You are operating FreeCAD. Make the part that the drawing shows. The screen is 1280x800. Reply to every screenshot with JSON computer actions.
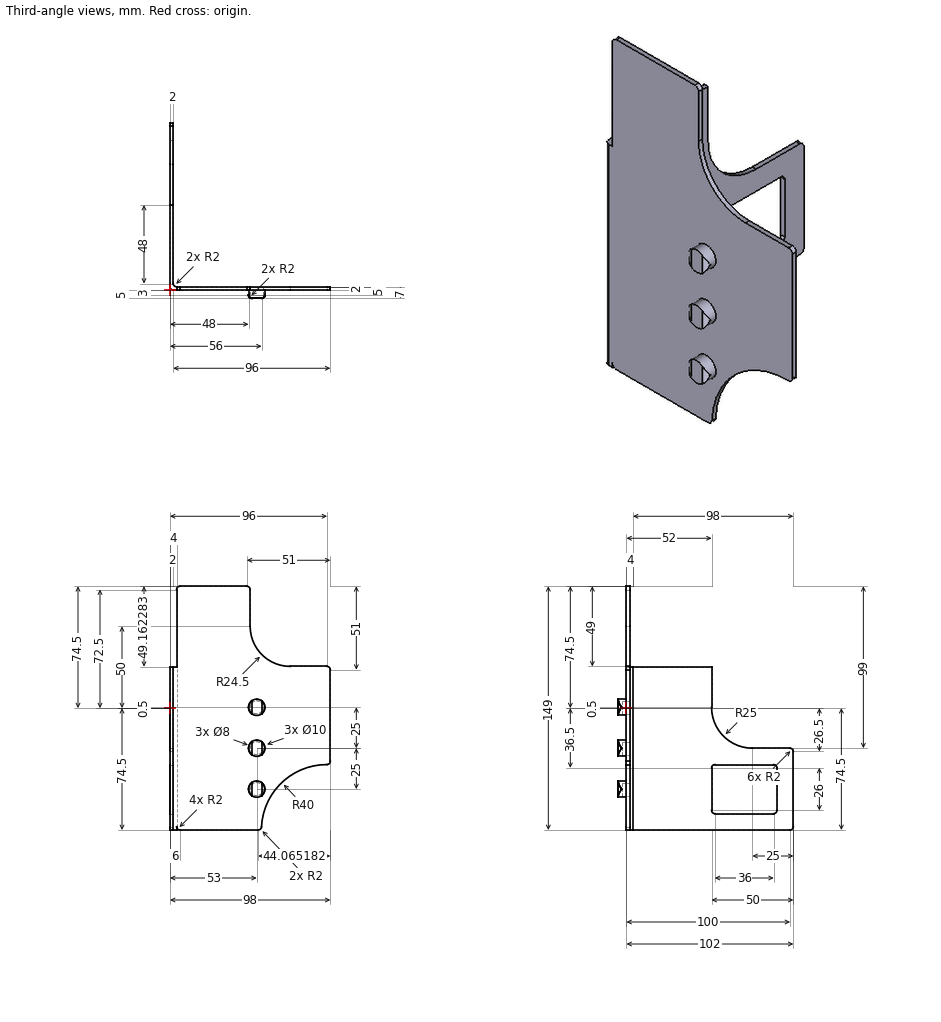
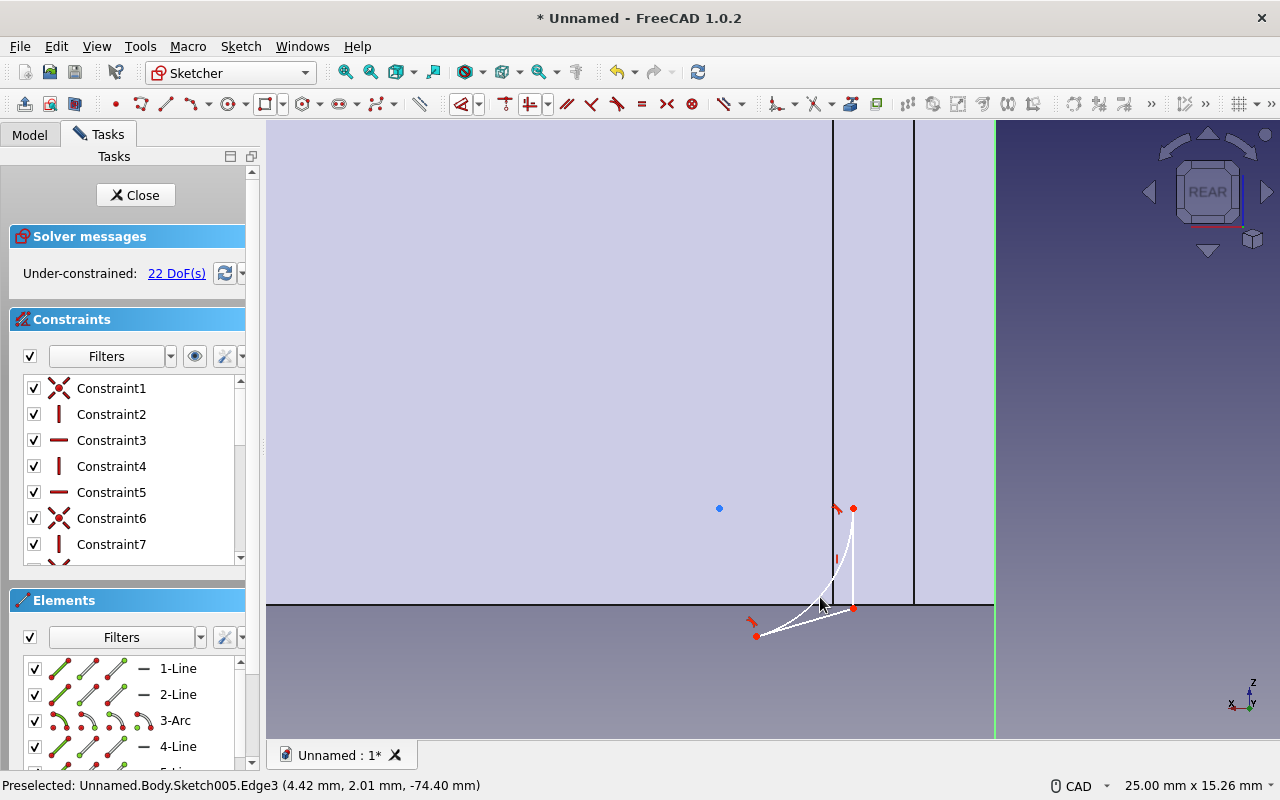
{"action": "scroll", "coordinate": [814, 614], "scroll_direction": "down", "scroll_amount": 14}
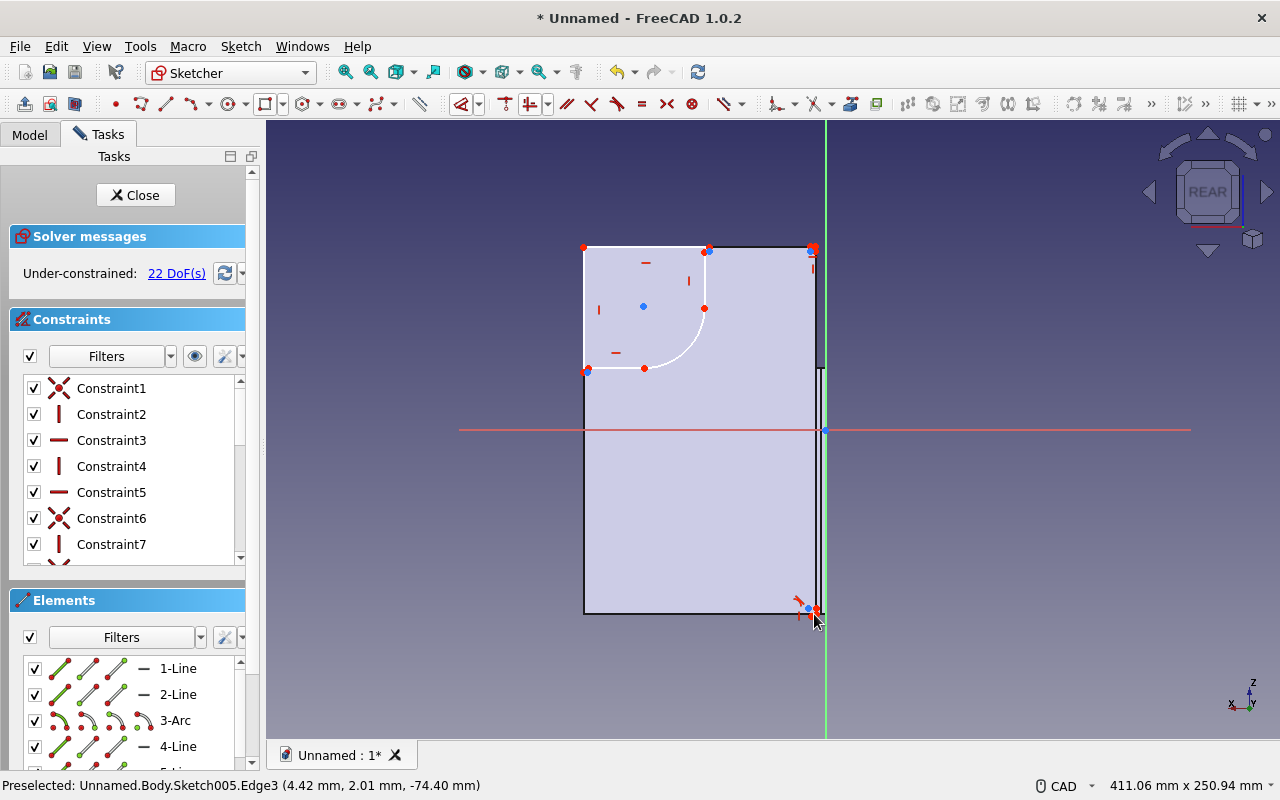
{"action": "left_click", "coordinate": [605, 368]}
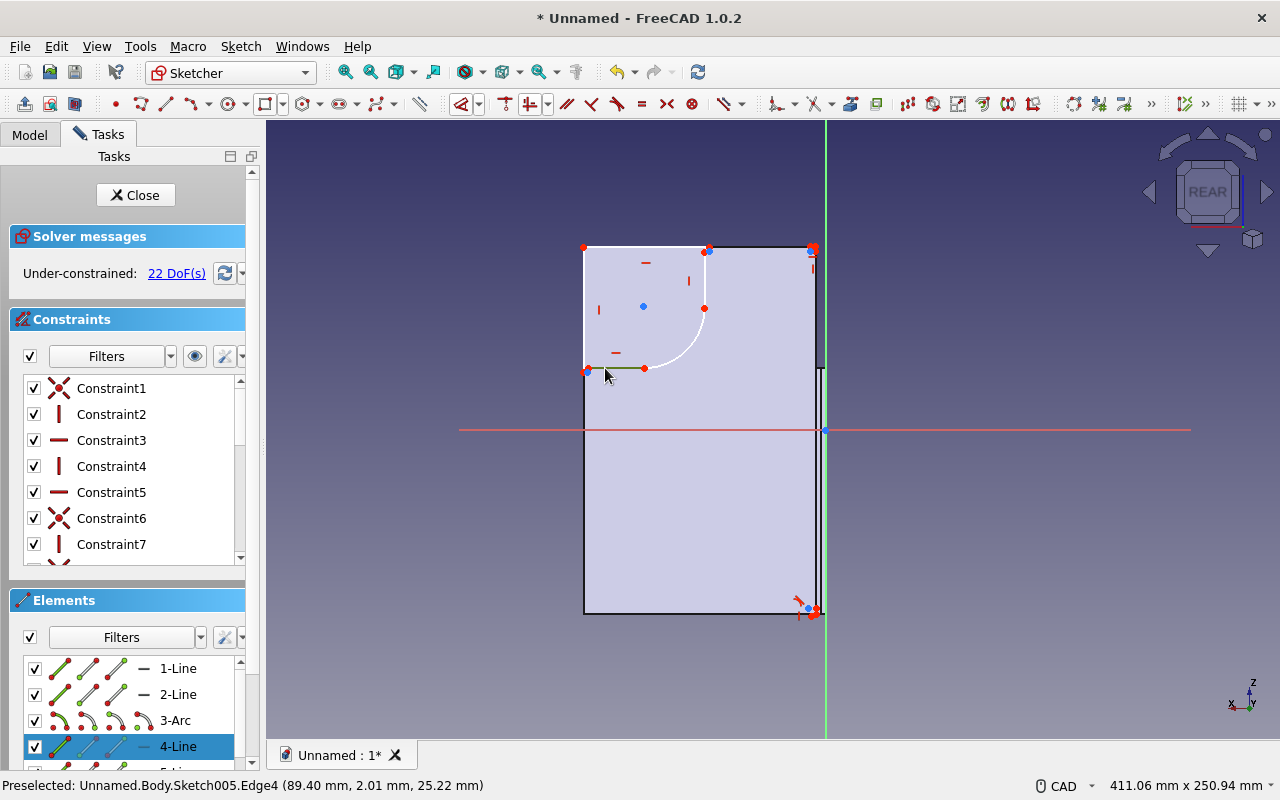
{"action": "left_click", "coordinate": [672, 361]}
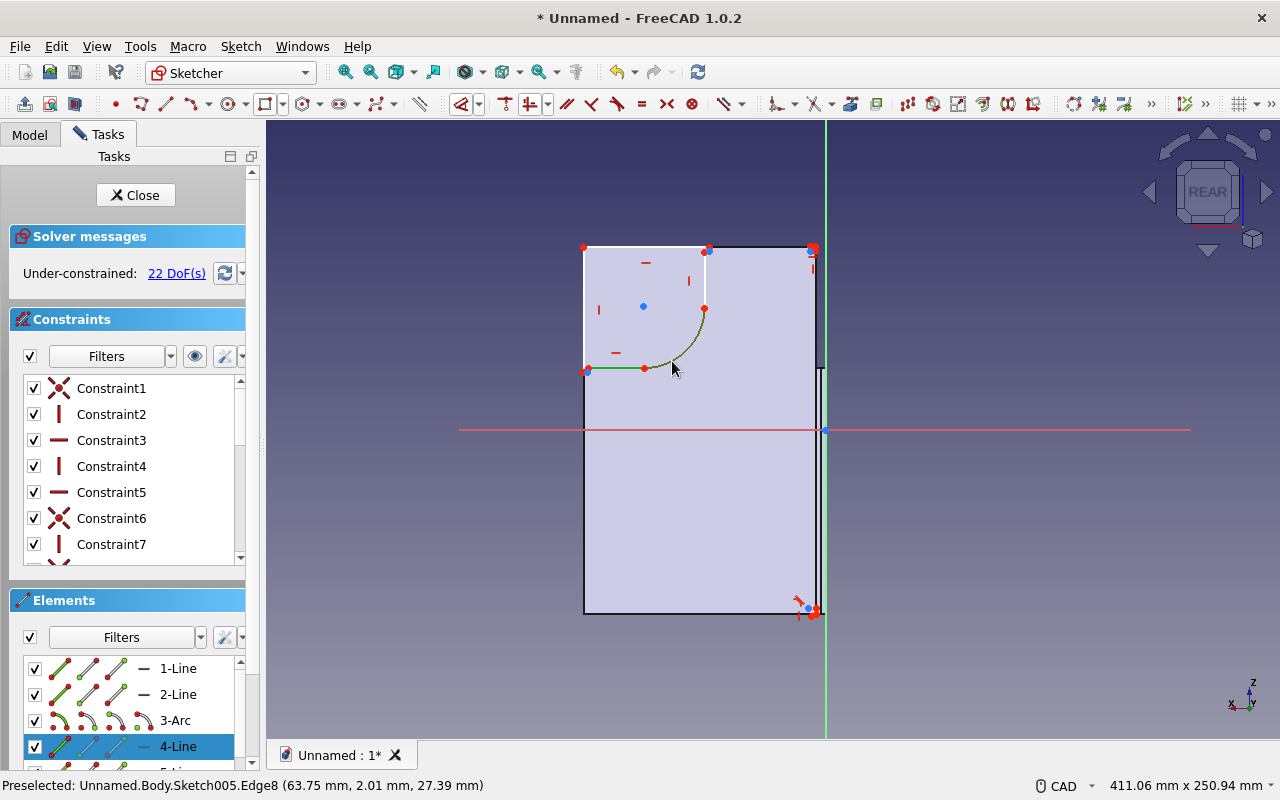
{"action": "key", "text": "t"}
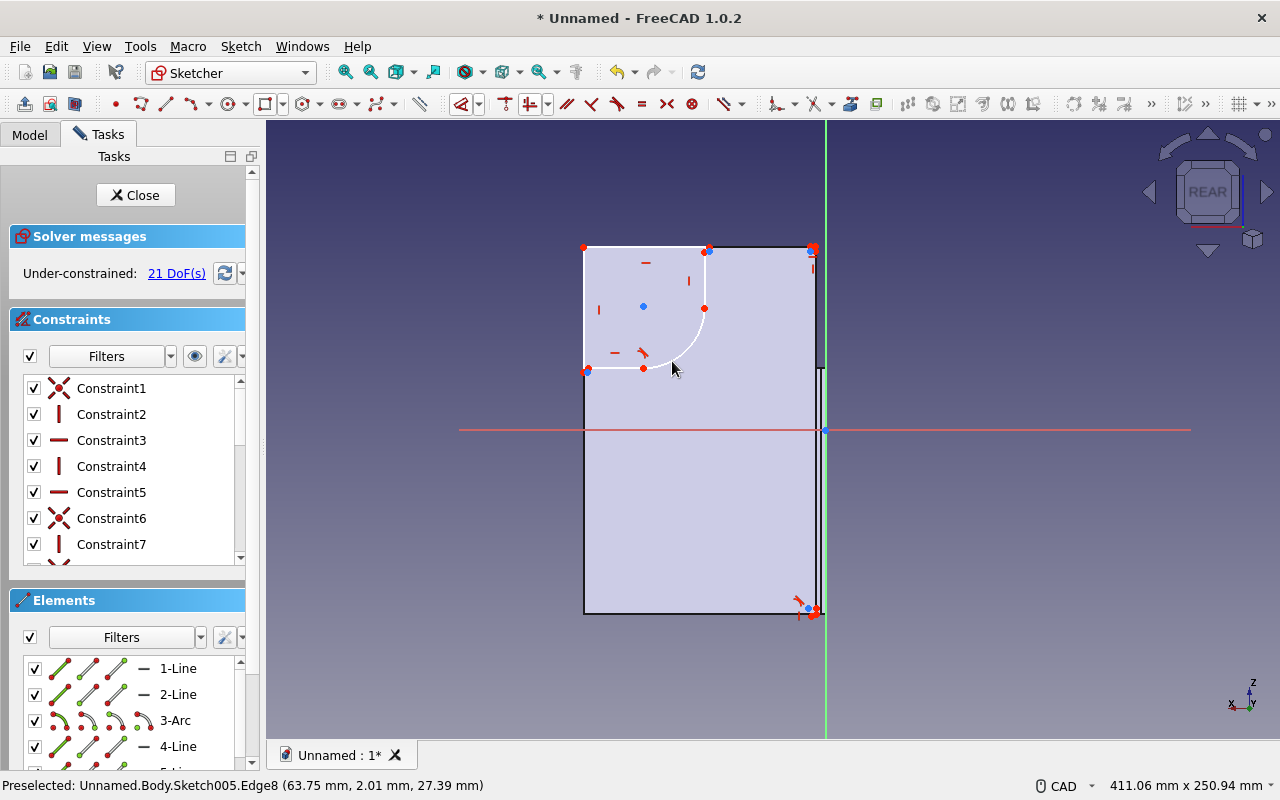
{"action": "left_click", "coordinate": [605, 368]}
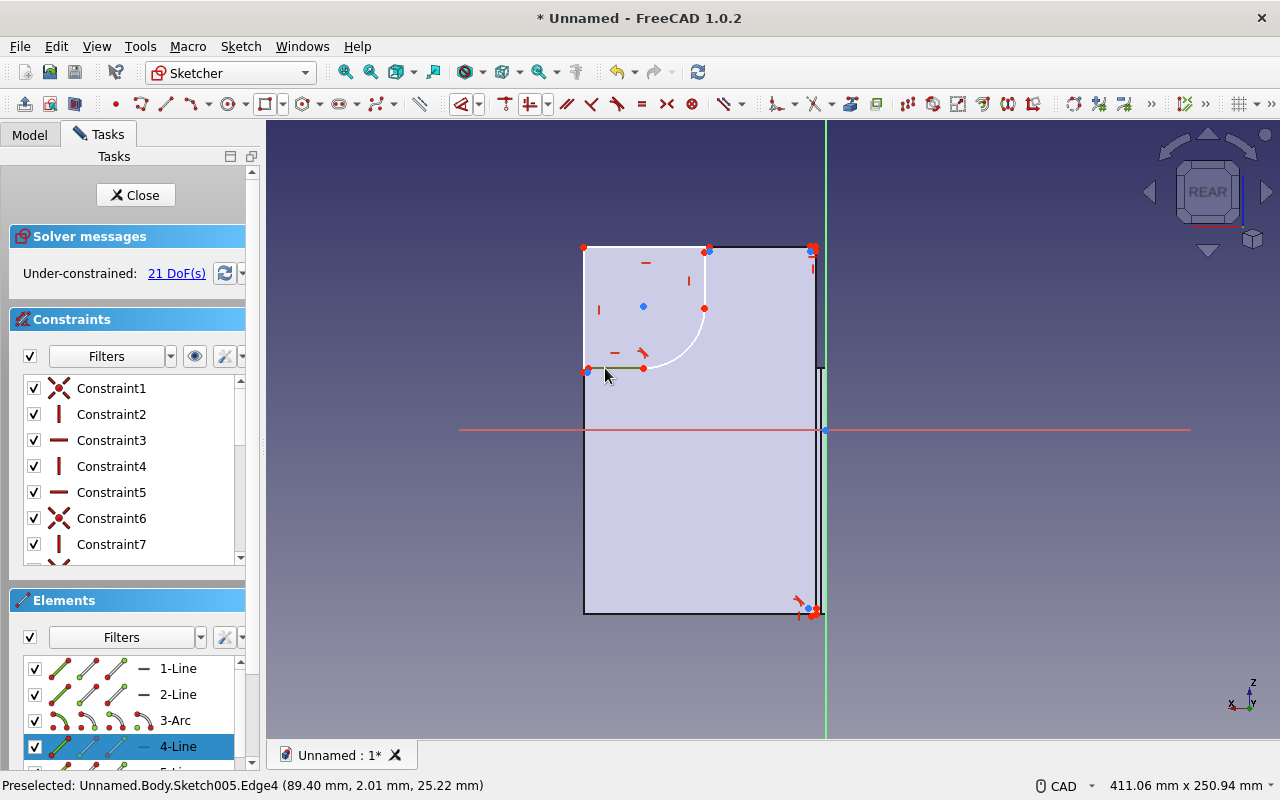
{"action": "scroll", "coordinate": [586, 368], "scroll_direction": "up", "scroll_amount": 9}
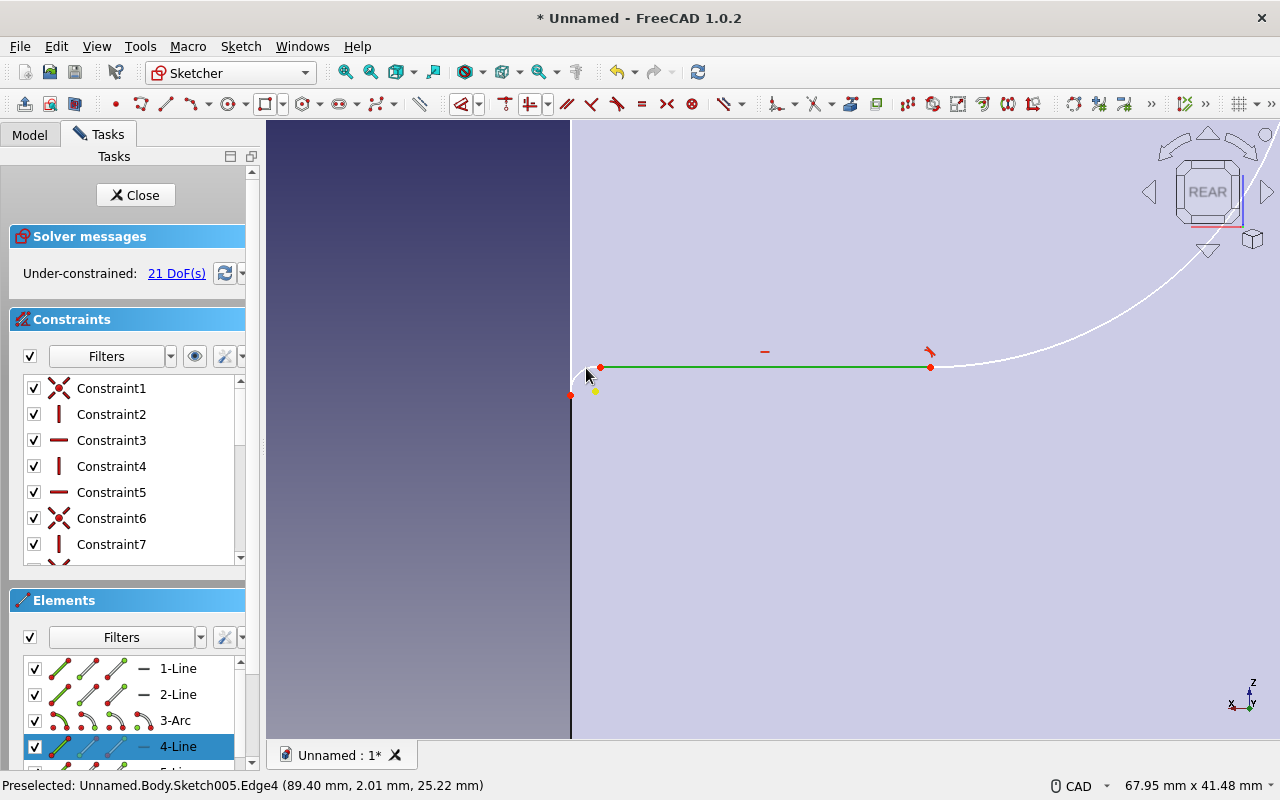
{"action": "left_click", "coordinate": [586, 369]}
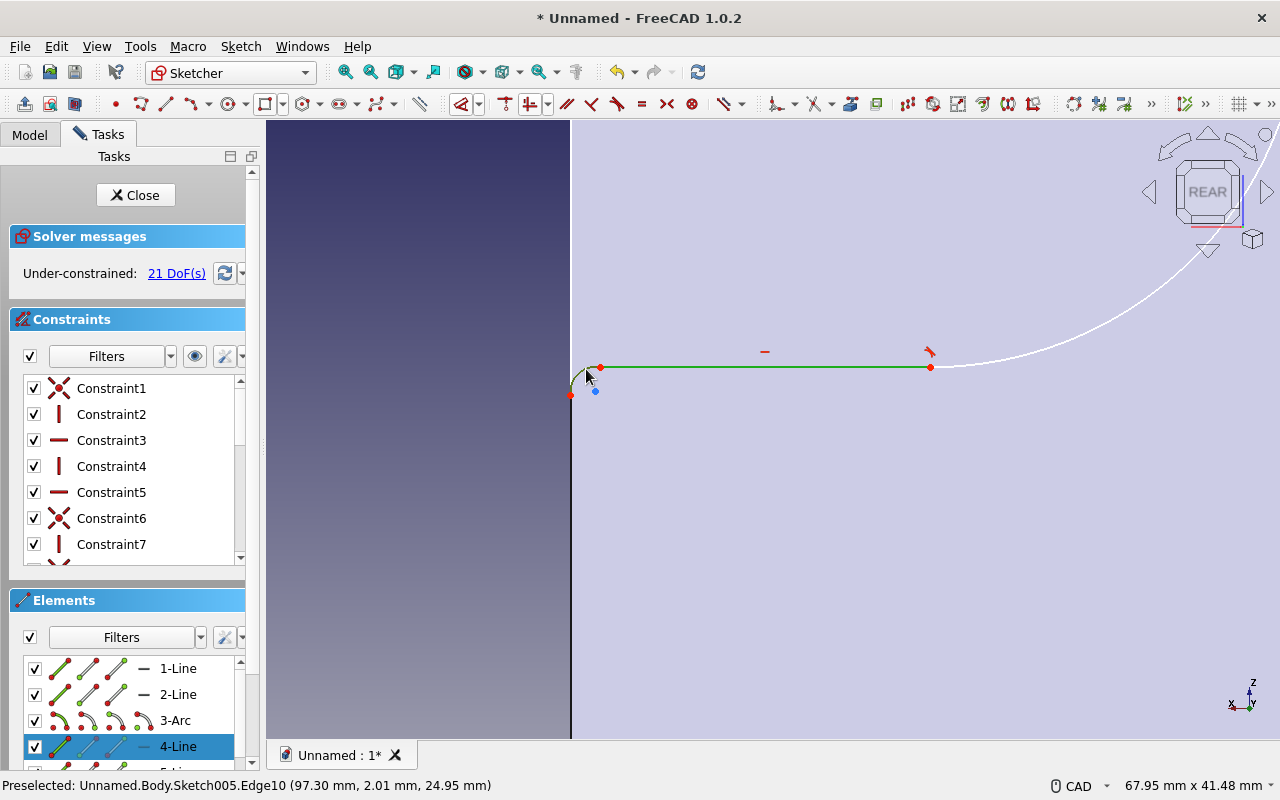
{"action": "key", "text": "t"}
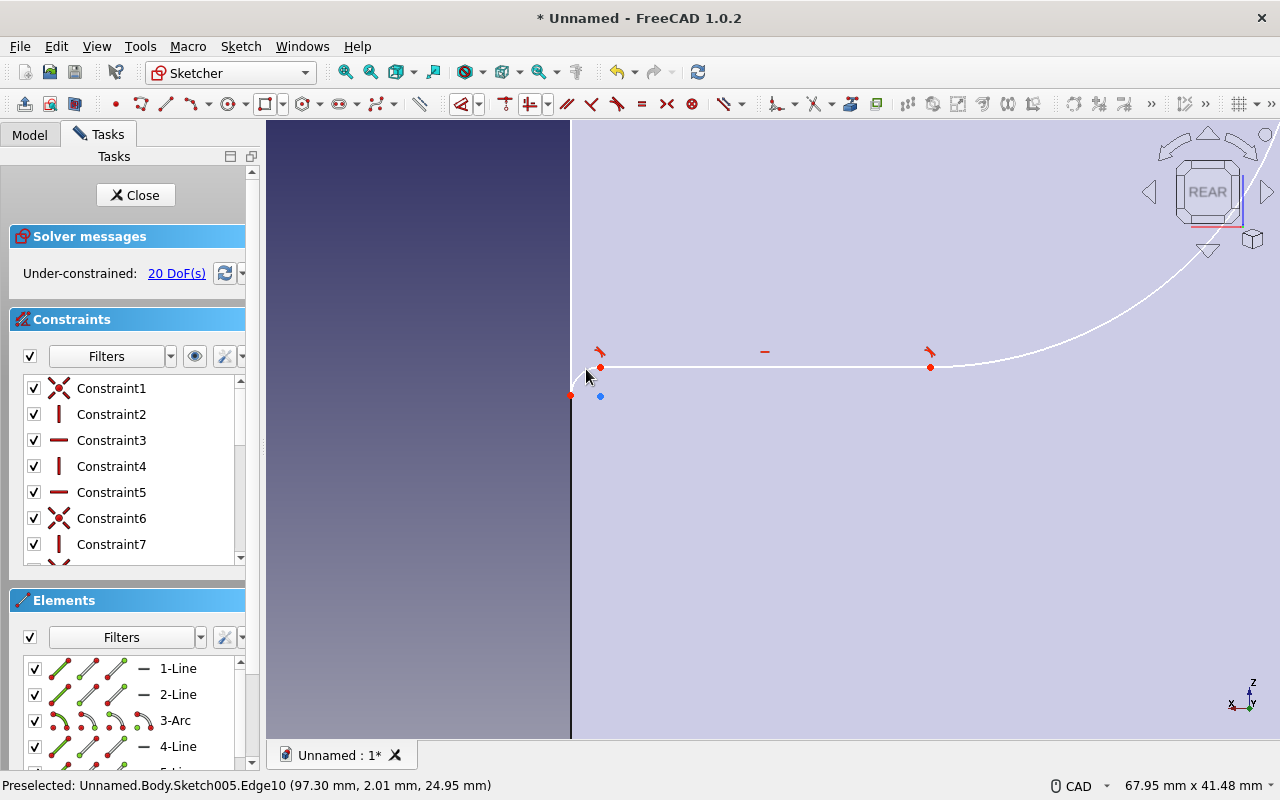
{"action": "scroll", "coordinate": [586, 367], "scroll_direction": "down", "scroll_amount": 9}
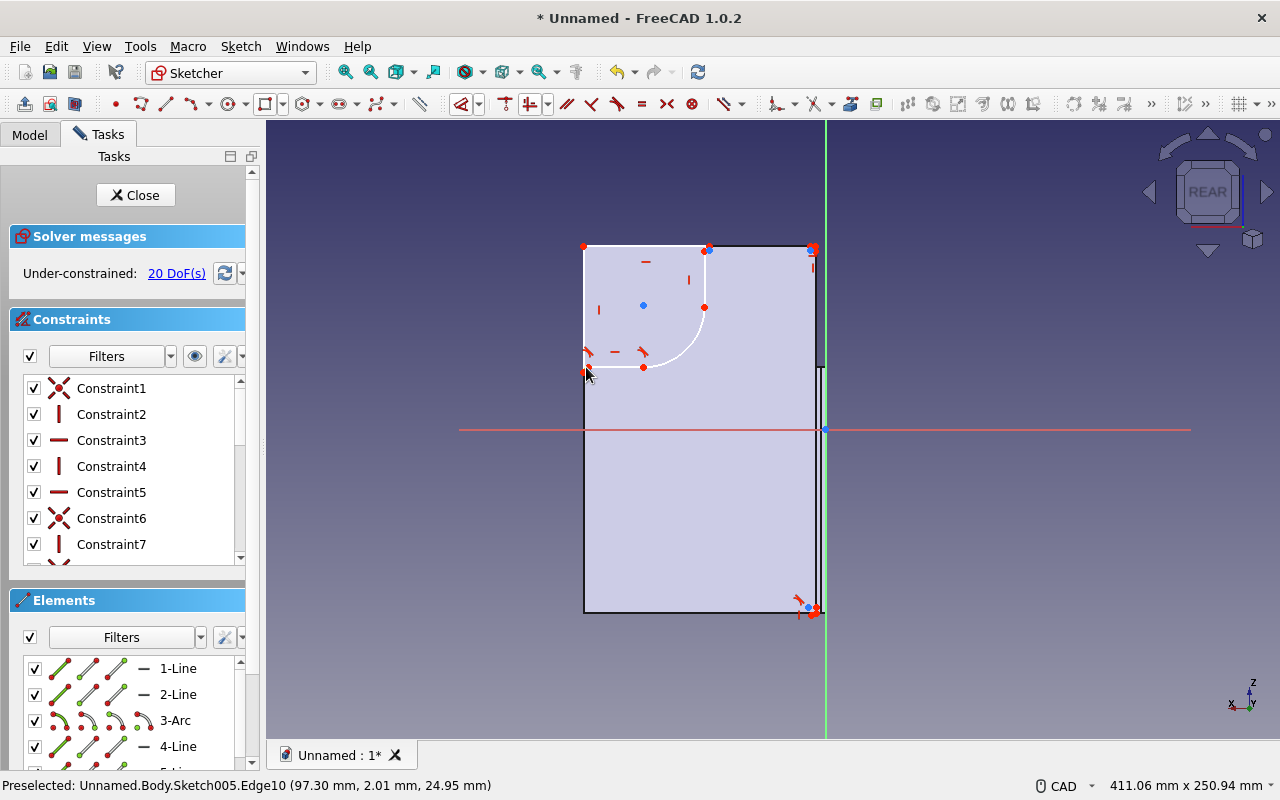
{"action": "left_click", "coordinate": [705, 291]}